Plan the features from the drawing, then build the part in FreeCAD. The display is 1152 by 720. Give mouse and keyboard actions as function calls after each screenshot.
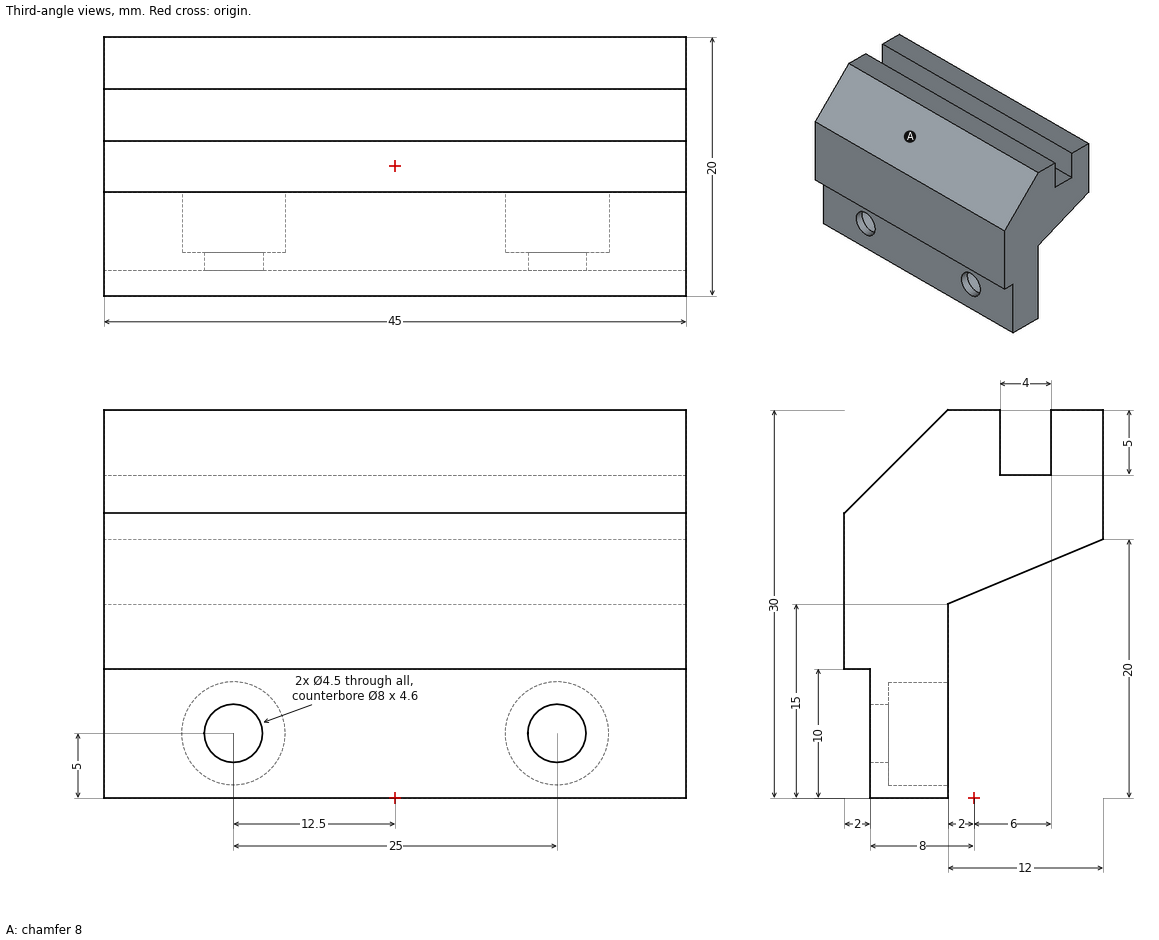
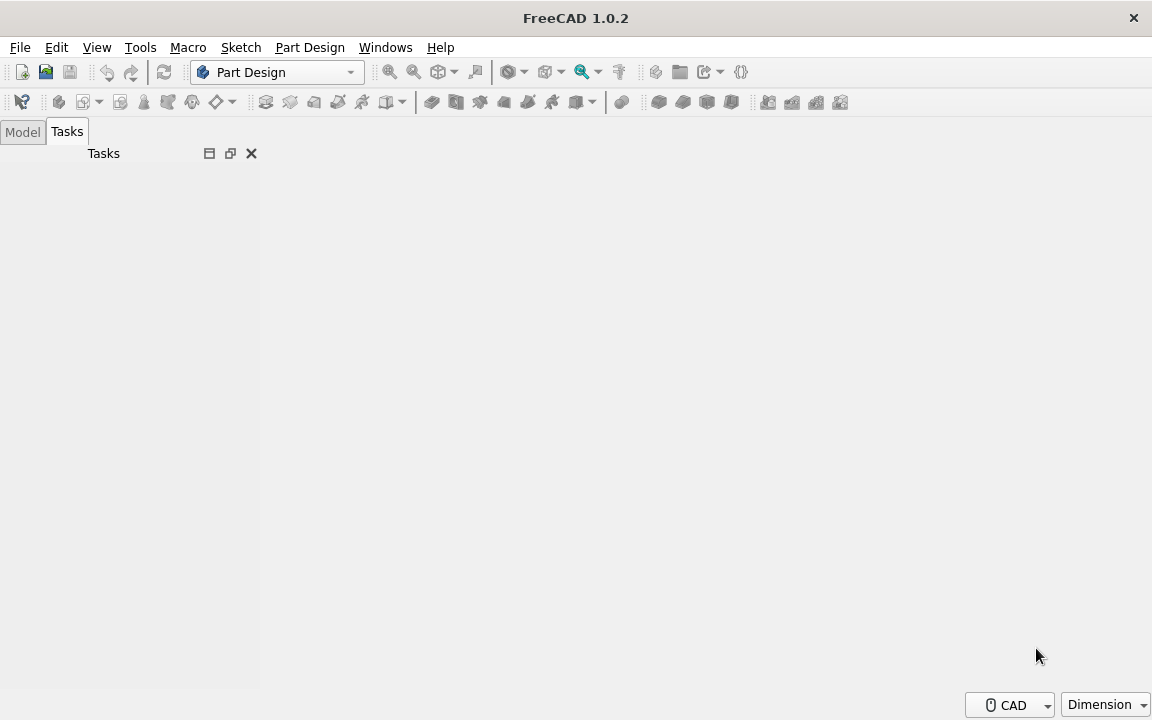
click(22, 72)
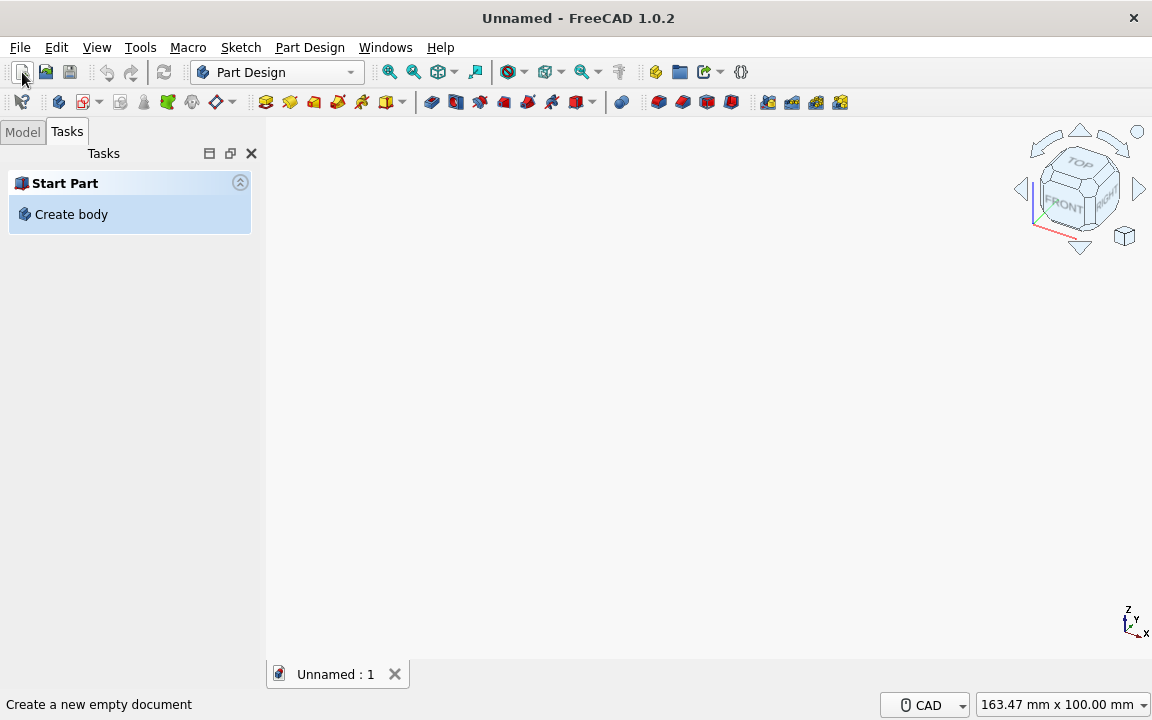
click(84, 102)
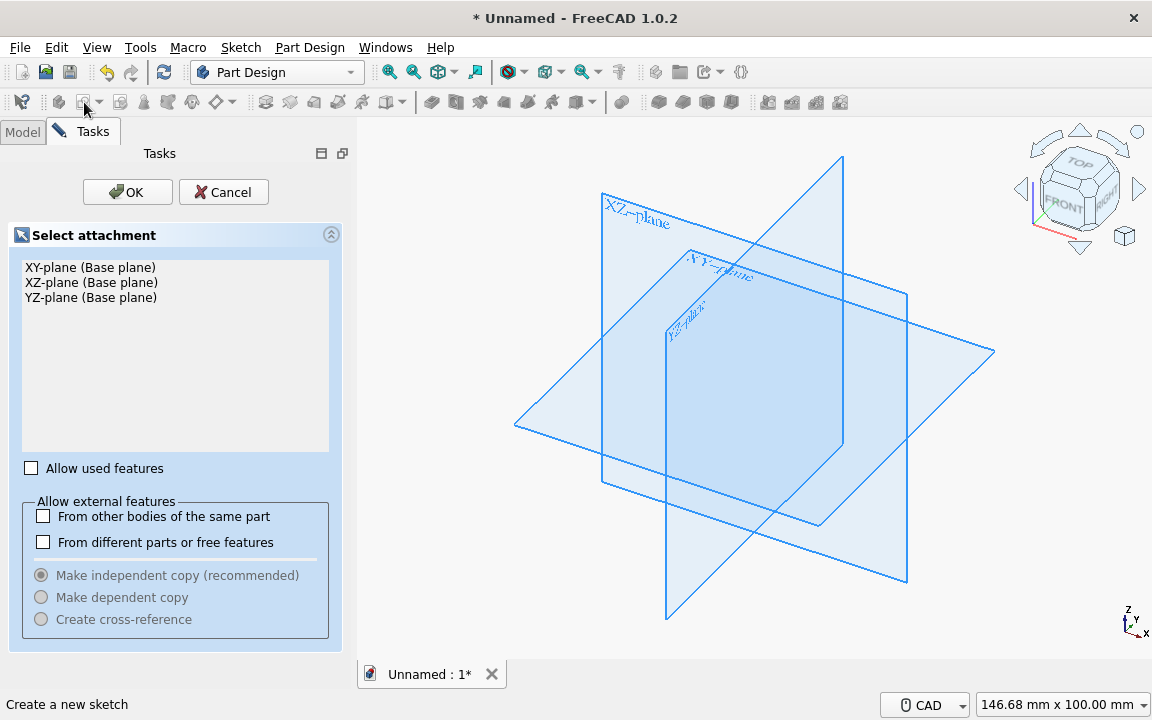
click(82, 268)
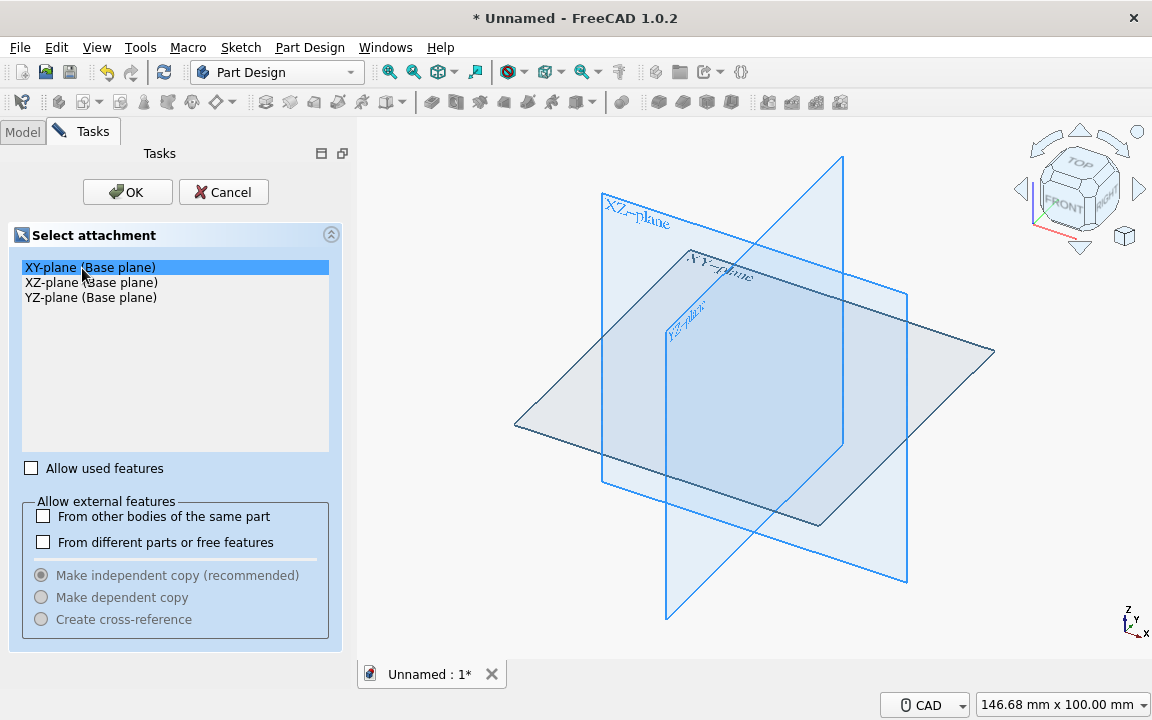
click(128, 192)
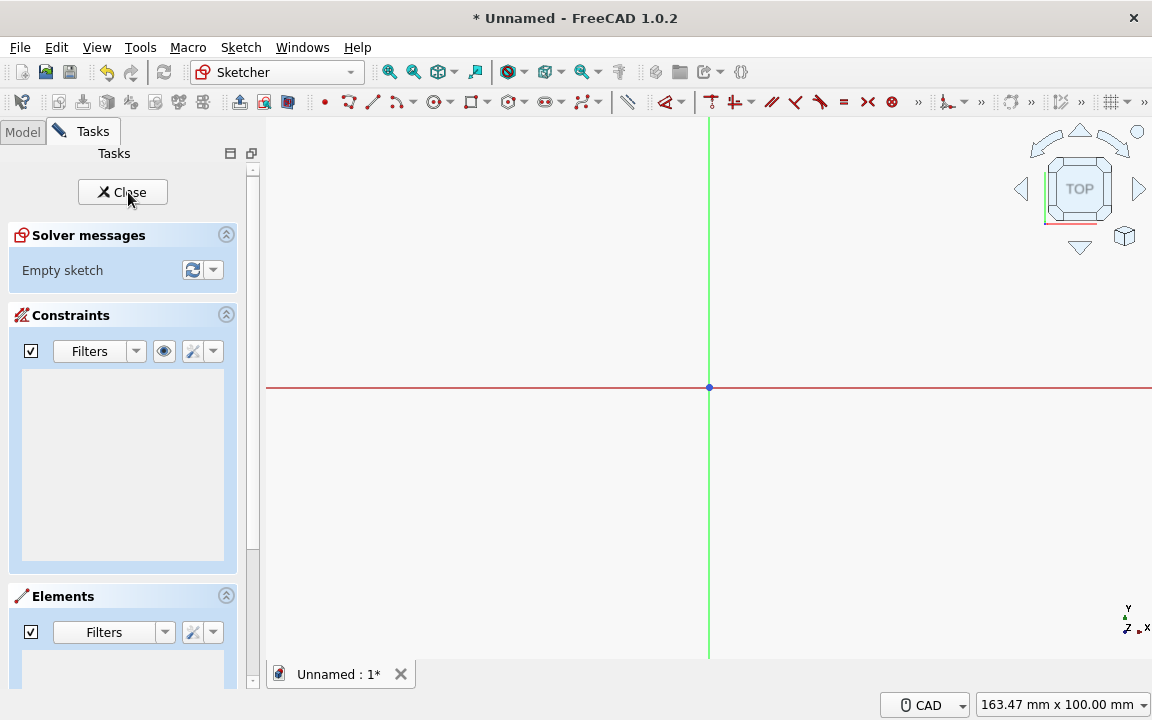
scroll(792, 388, up, 3)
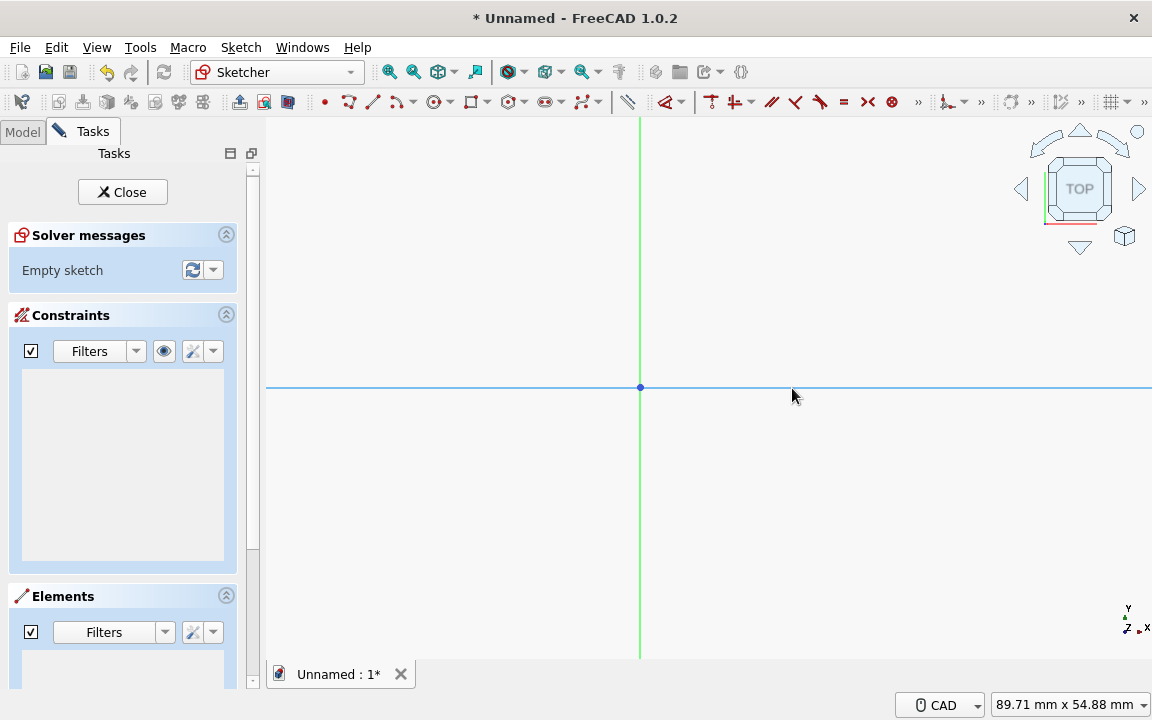
key(g)
key(v)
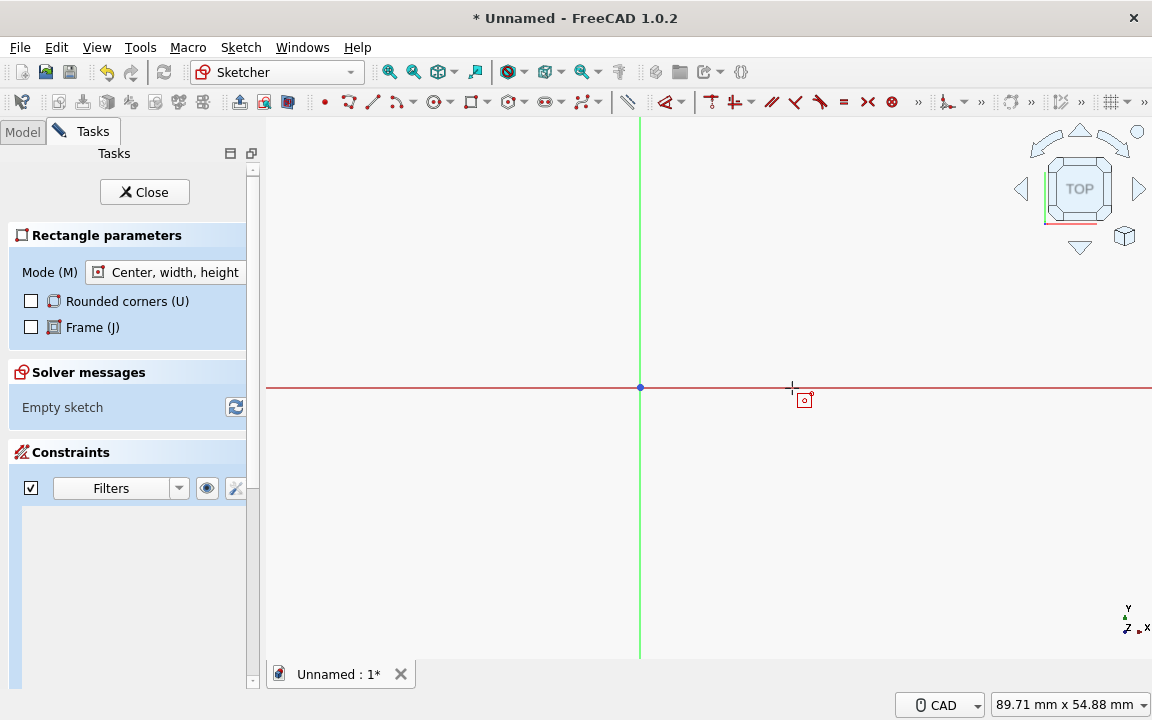
click(640, 388)
move(862, 289)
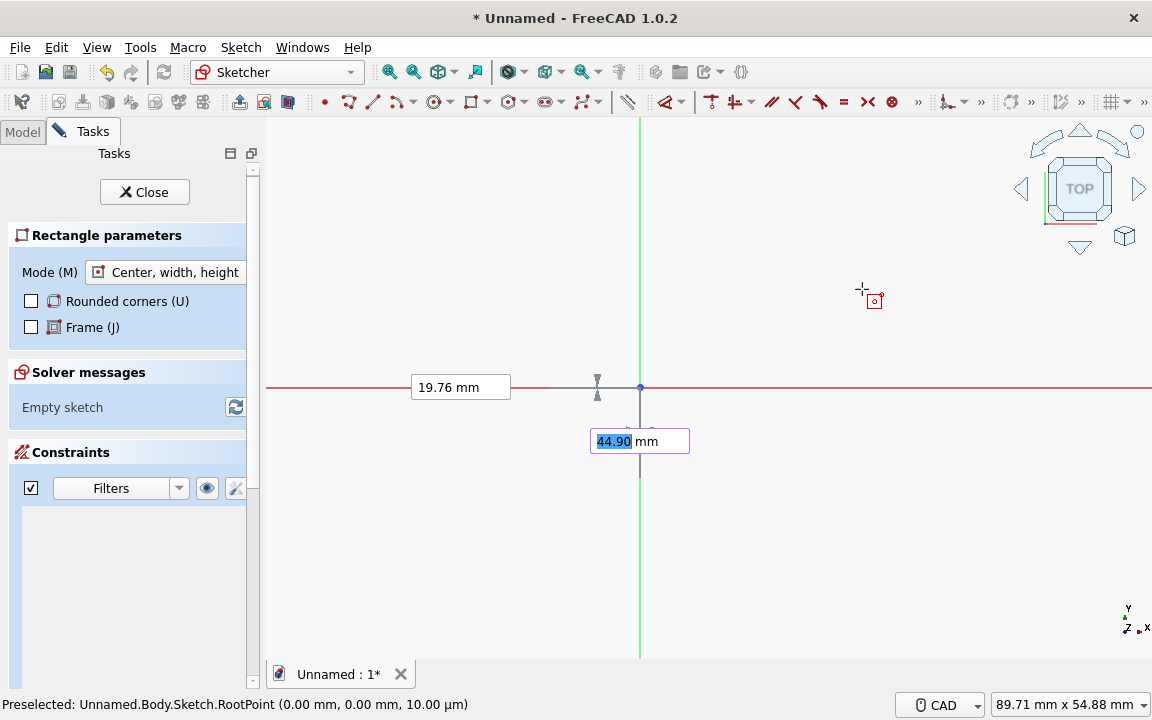
text(45)
key(Tab)
text(20)
key(Return)
key(Escape)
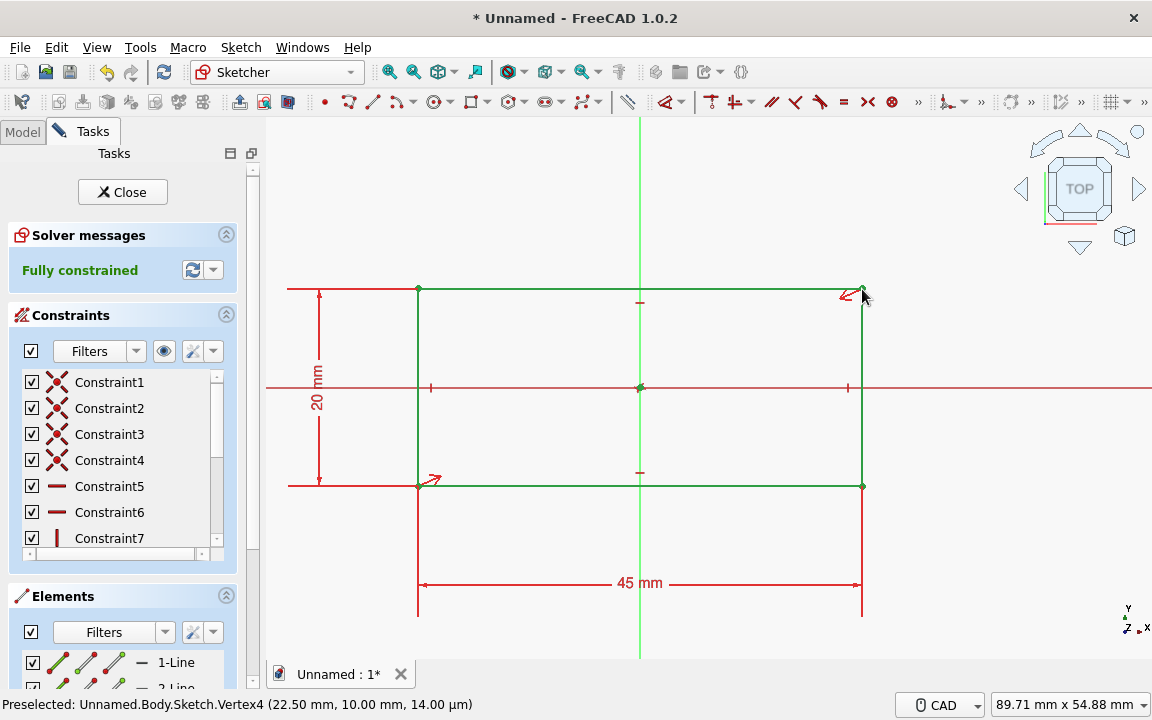
click(123, 192)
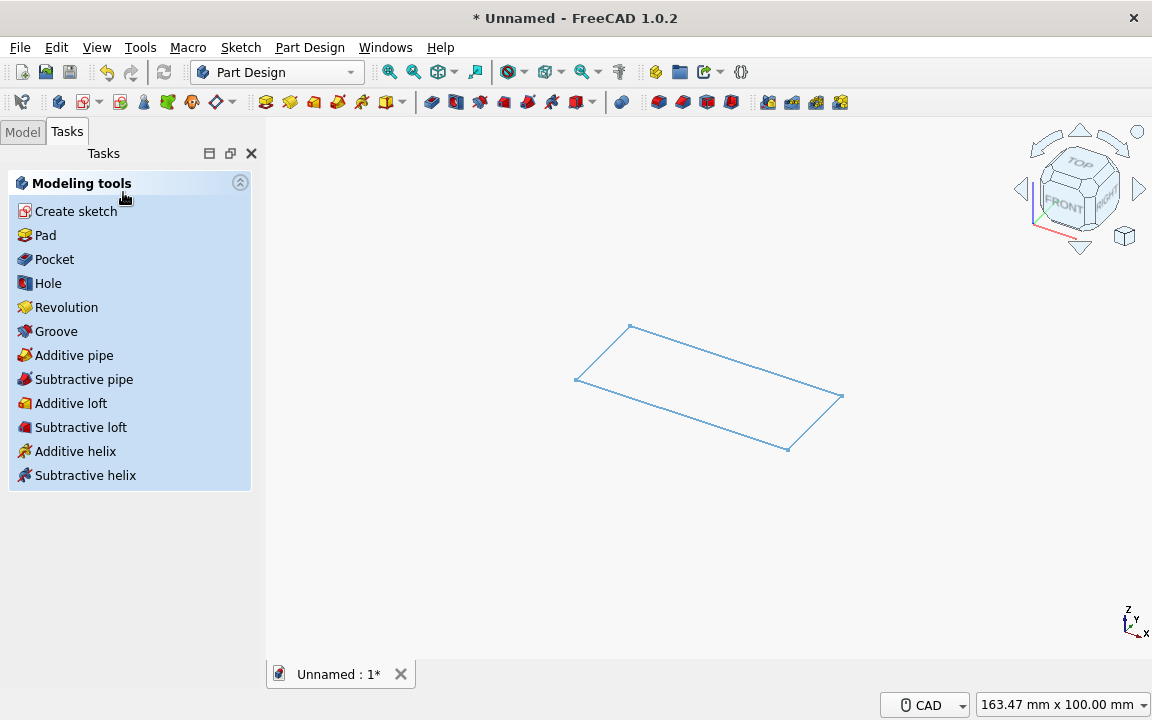
click(266, 102)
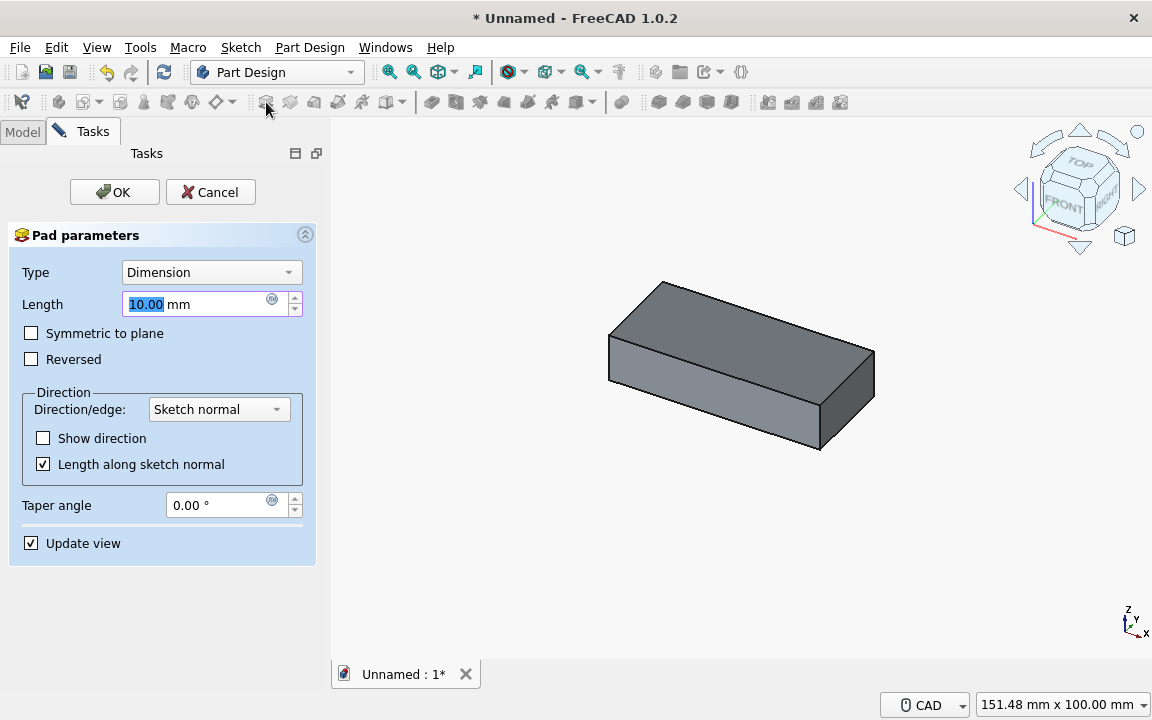
text(30)
key(Tab)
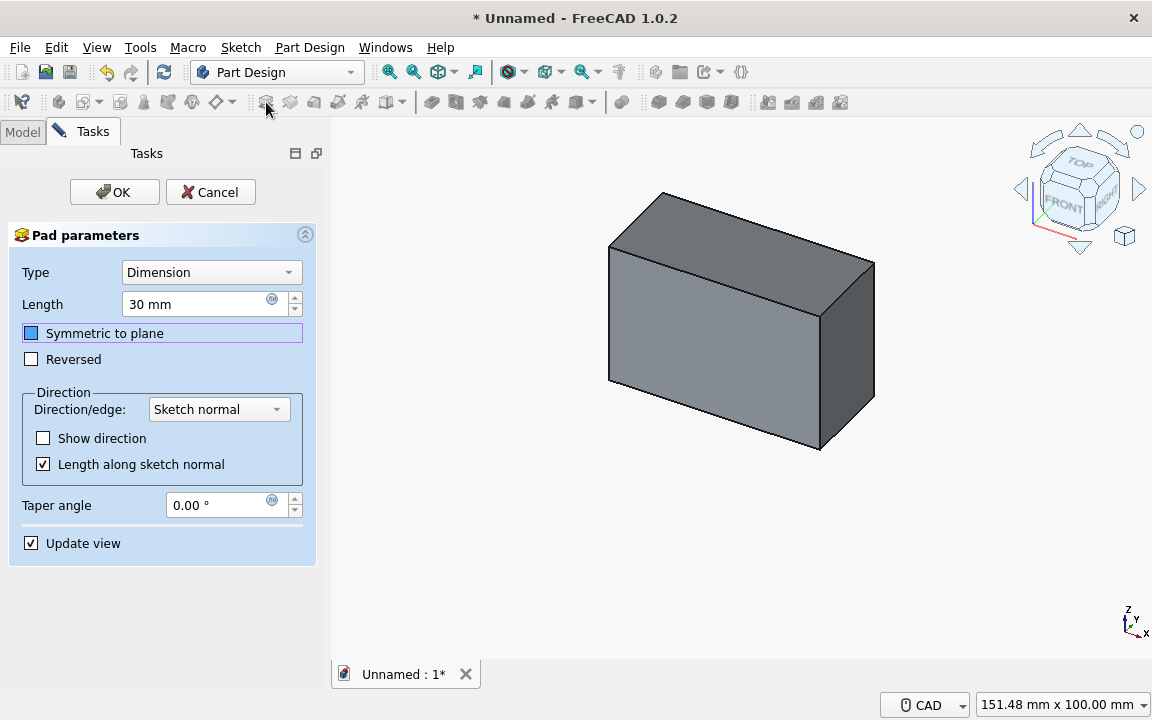
click(115, 192)